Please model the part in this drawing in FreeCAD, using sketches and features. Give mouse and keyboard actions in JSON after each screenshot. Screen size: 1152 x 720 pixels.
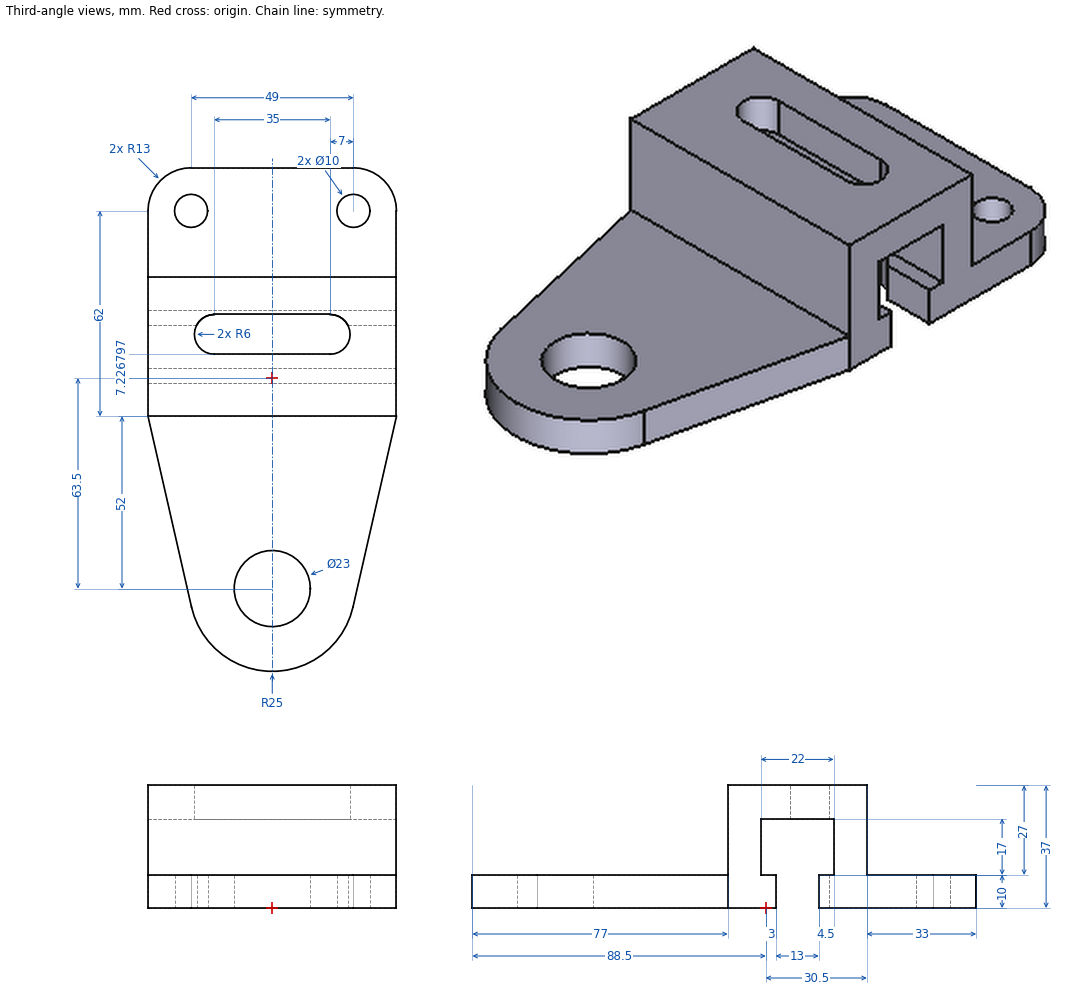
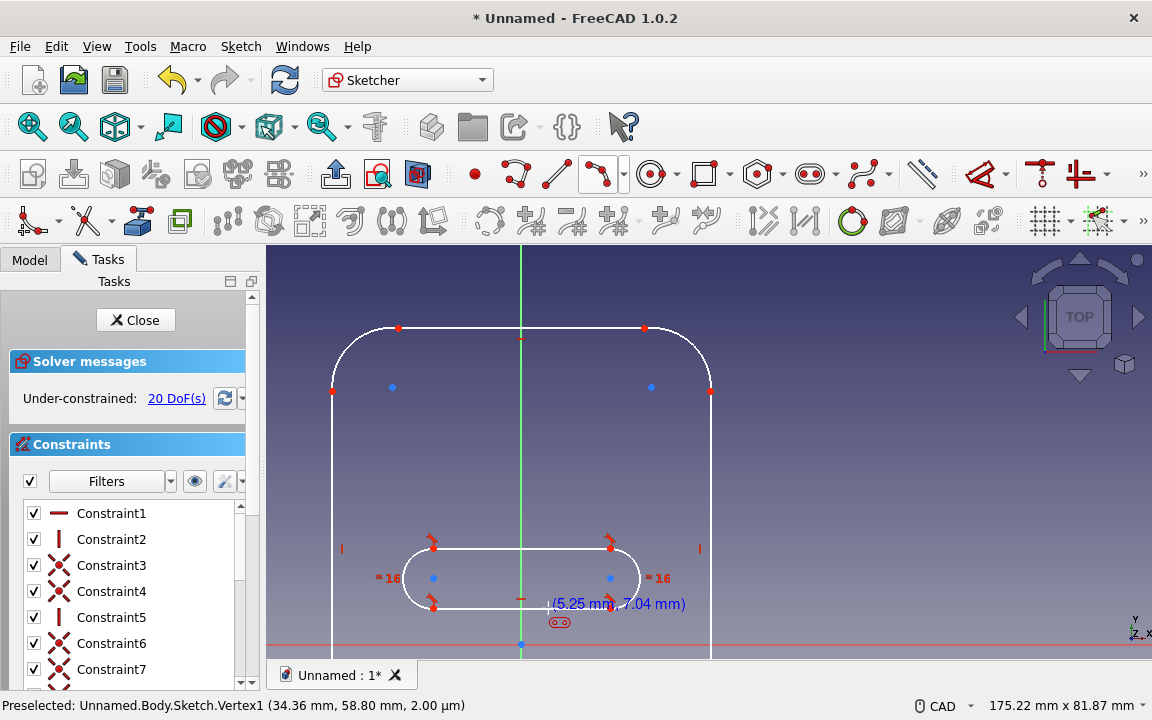
{"action": "left_click", "coordinate": [650, 174]}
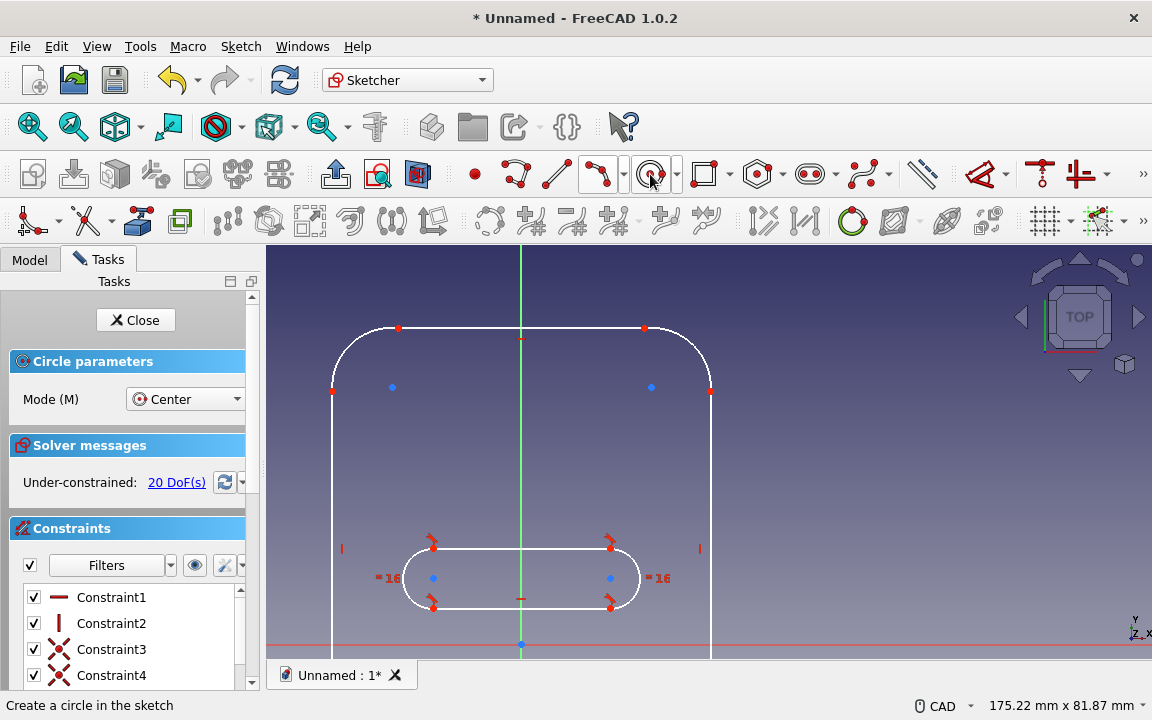
{"action": "scroll", "coordinate": [692, 342], "scroll_direction": "down", "scroll_amount": 6}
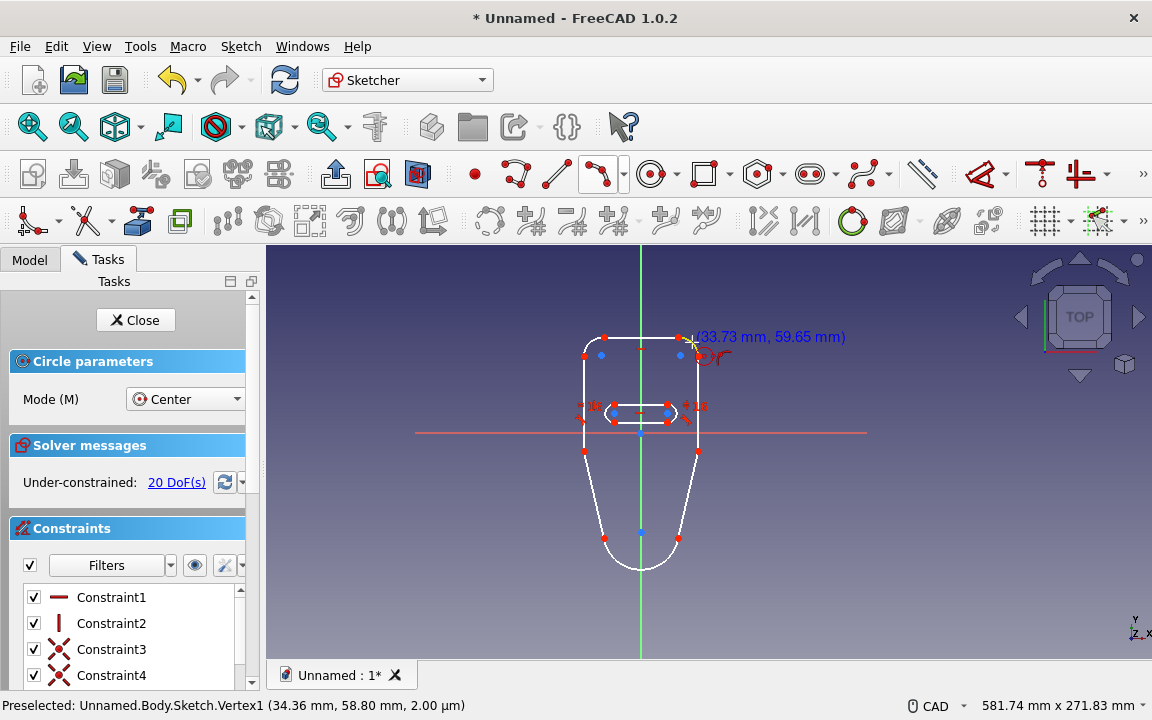
{"action": "scroll", "coordinate": [641, 530], "scroll_direction": "up", "scroll_amount": 2}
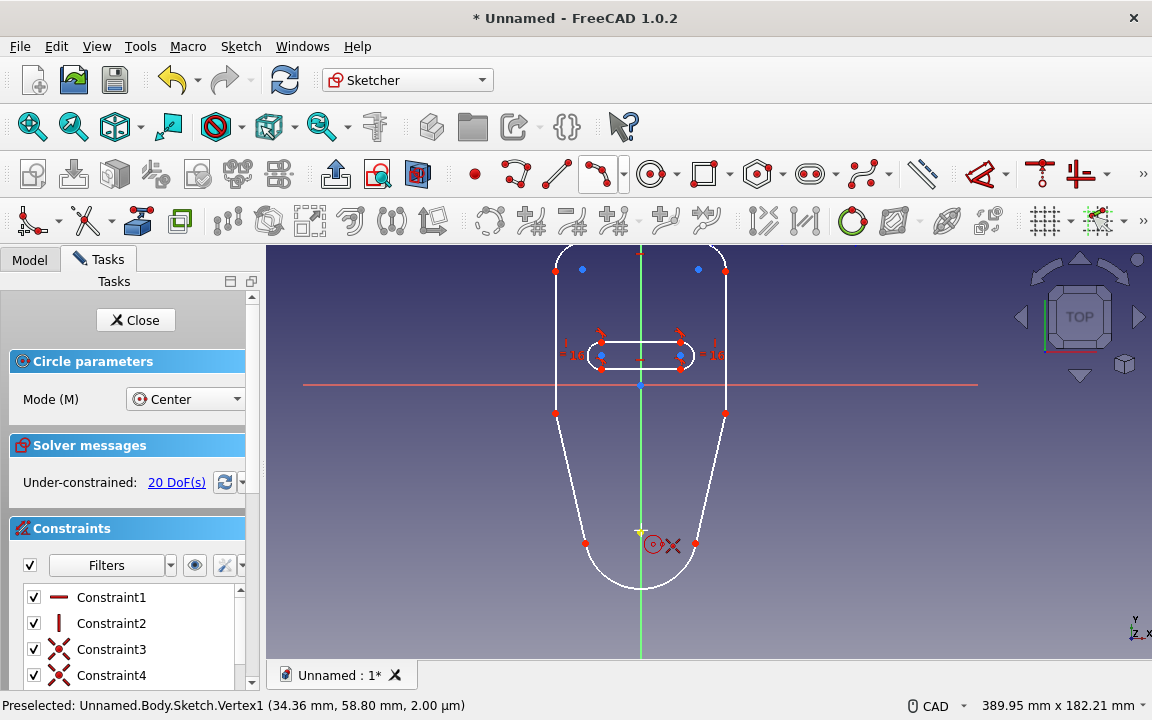
{"action": "left_click", "coordinate": [641, 530]}
{"action": "mouse_move", "coordinate": [659, 511]}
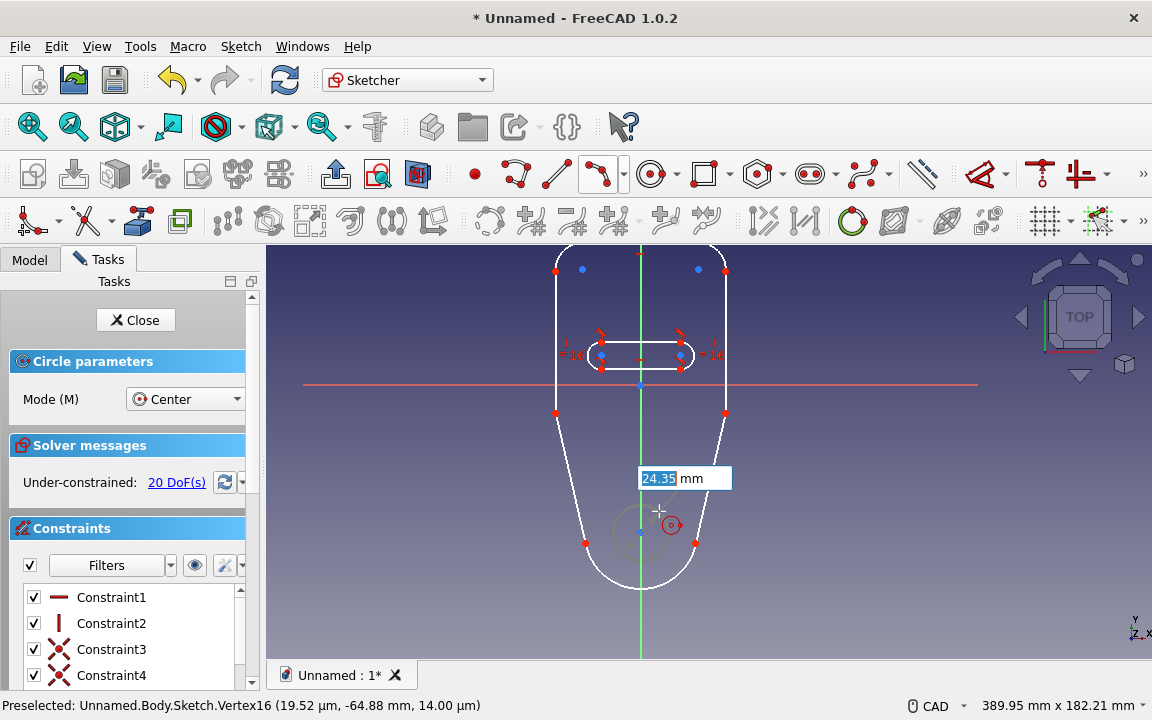
{"action": "type", "text": "23"}
{"action": "key", "text": "Return"}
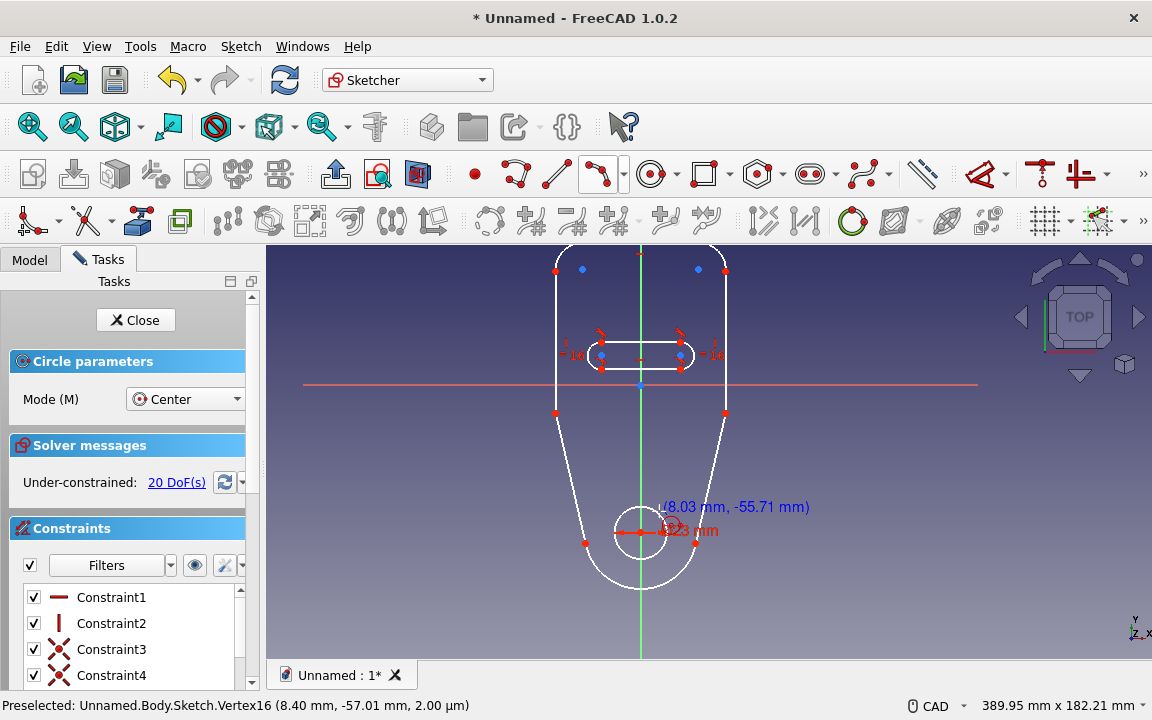
{"action": "scroll", "coordinate": [640, 530], "scroll_direction": "down", "scroll_amount": 2}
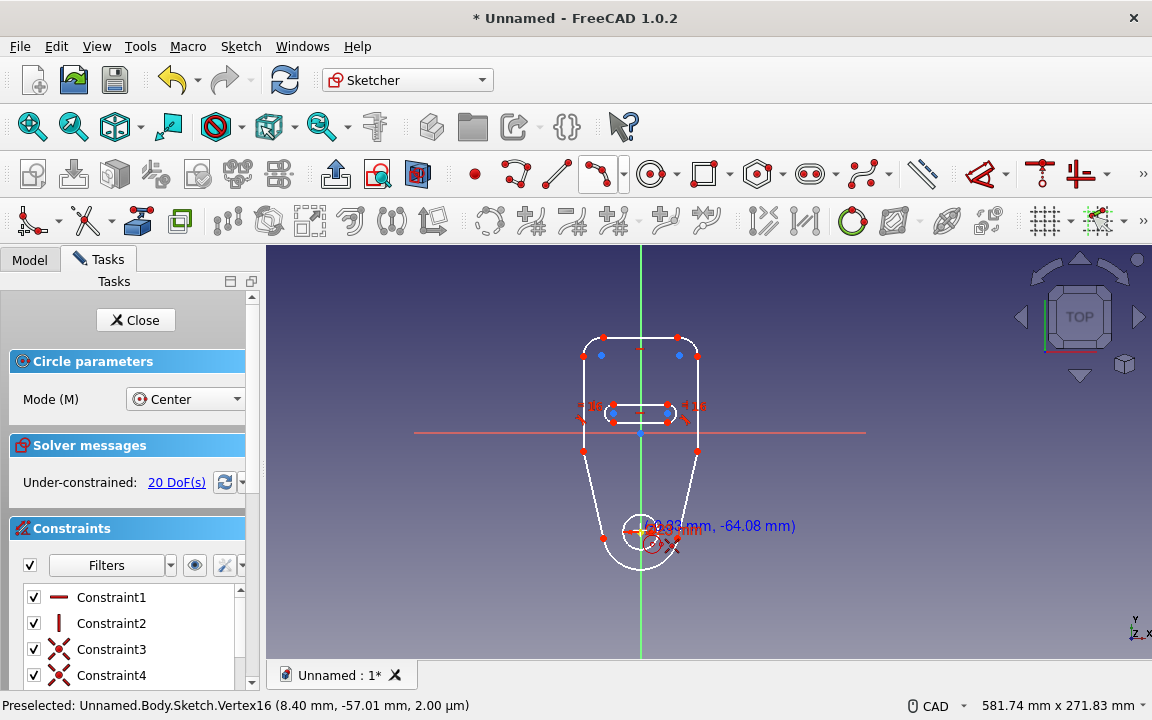
{"action": "scroll", "coordinate": [678, 356], "scroll_direction": "up", "scroll_amount": 6}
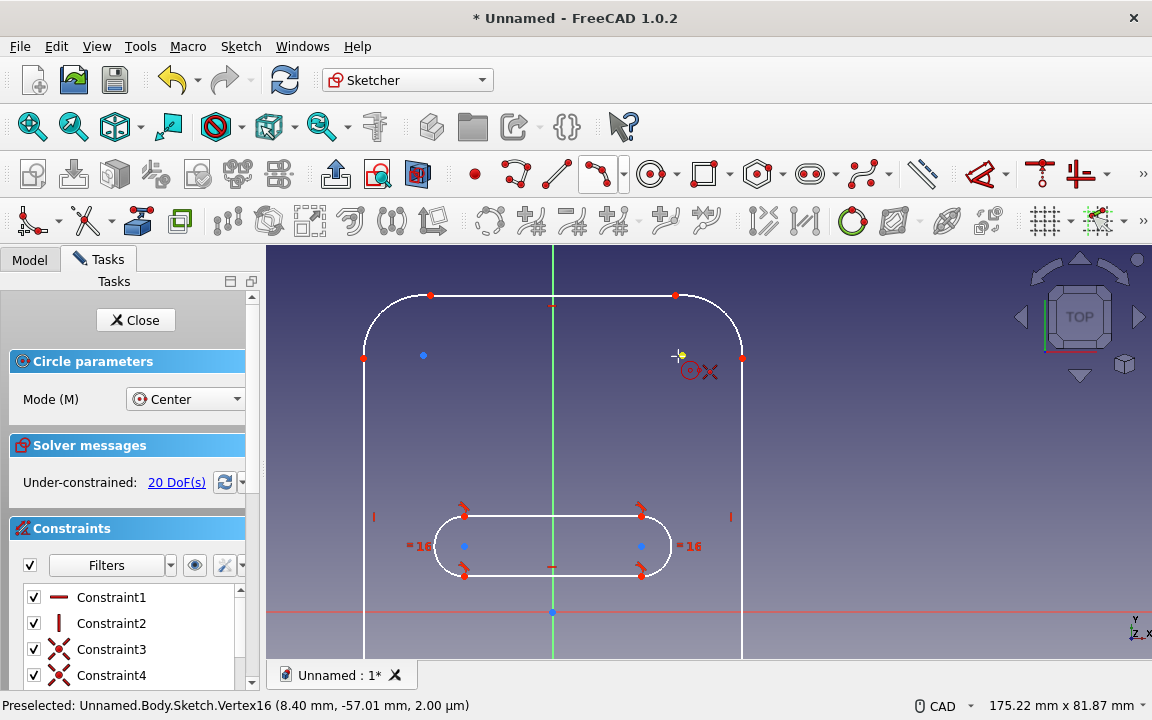
{"action": "left_click", "coordinate": [677, 357]}
{"action": "mouse_move", "coordinate": [695, 339]}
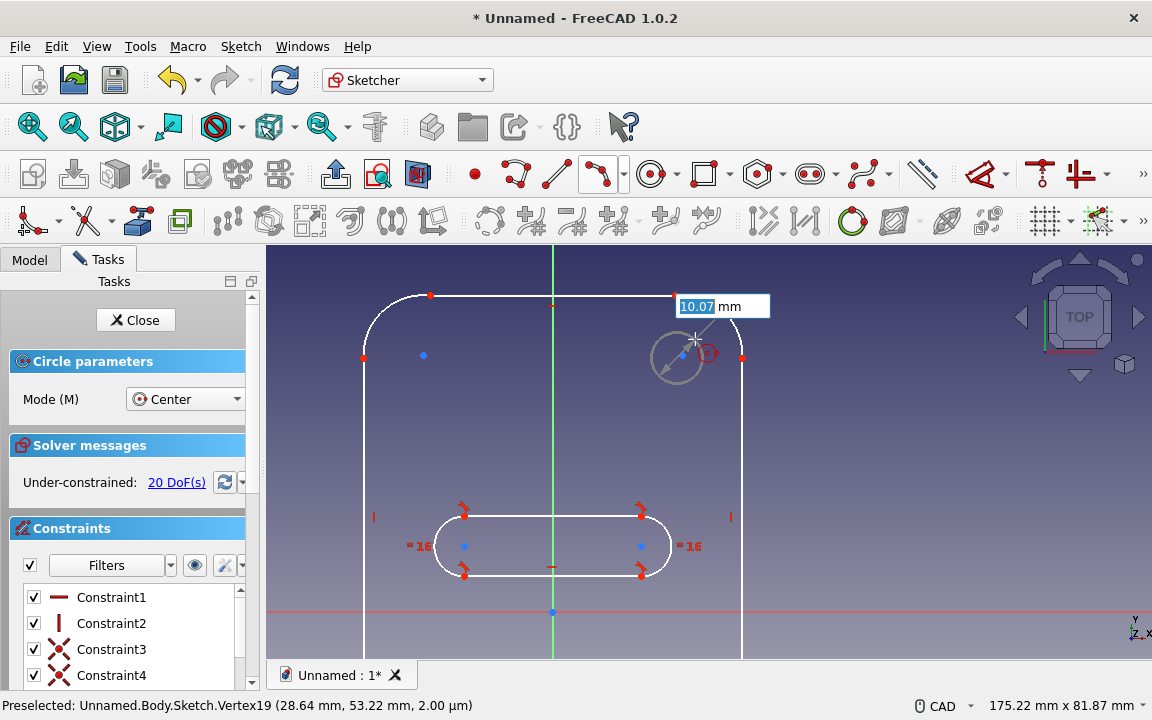
{"action": "type", "text": "10"}
{"action": "key", "text": "Return"}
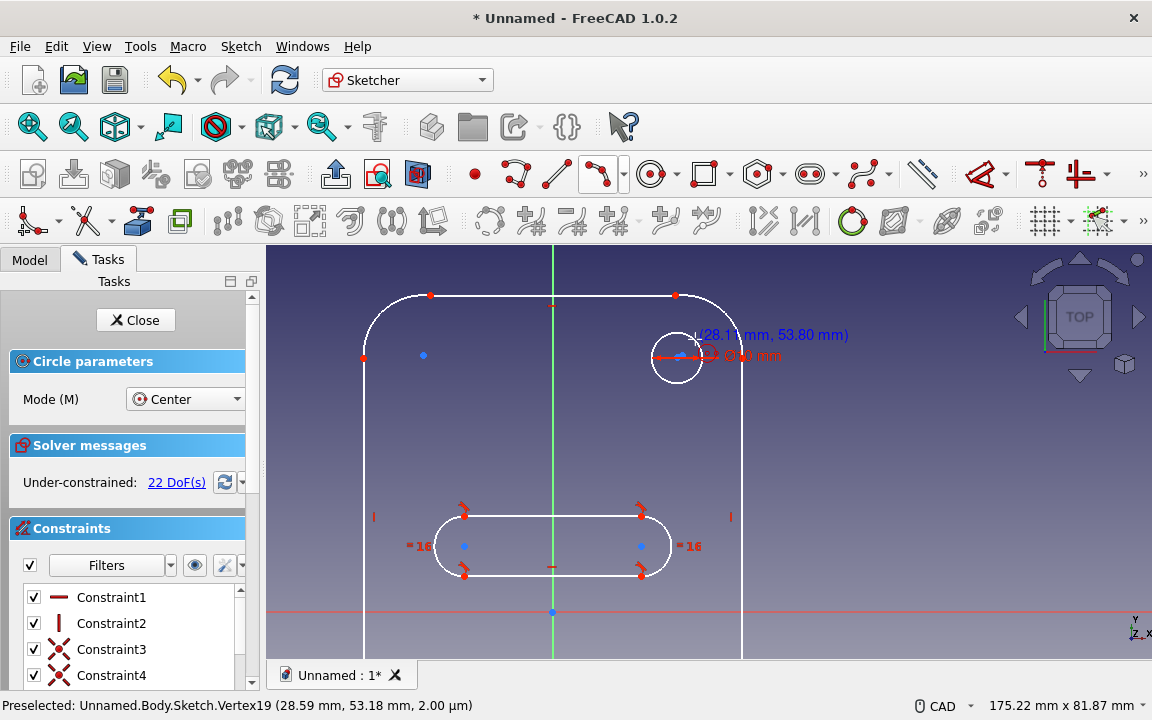
{"action": "left_click", "coordinate": [429, 357]}
{"action": "mouse_move", "coordinate": [447, 339]}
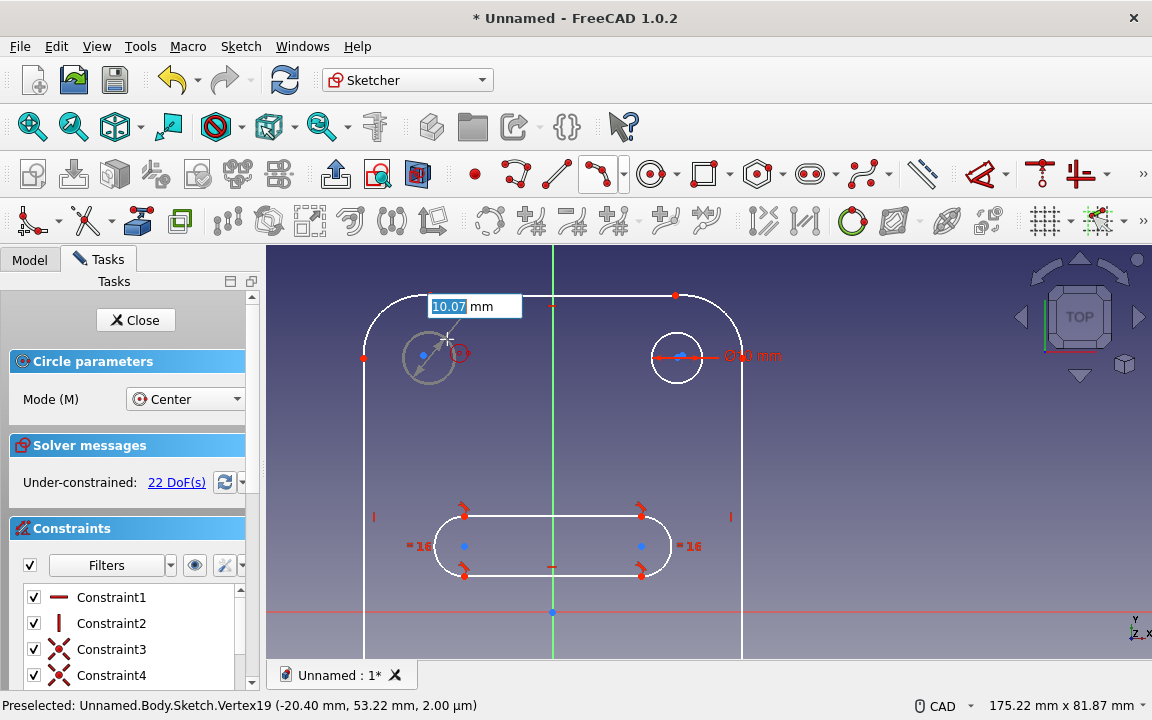
{"action": "type", "text": "10"}
{"action": "key", "text": "Return"}
{"action": "key", "text": "Escape"}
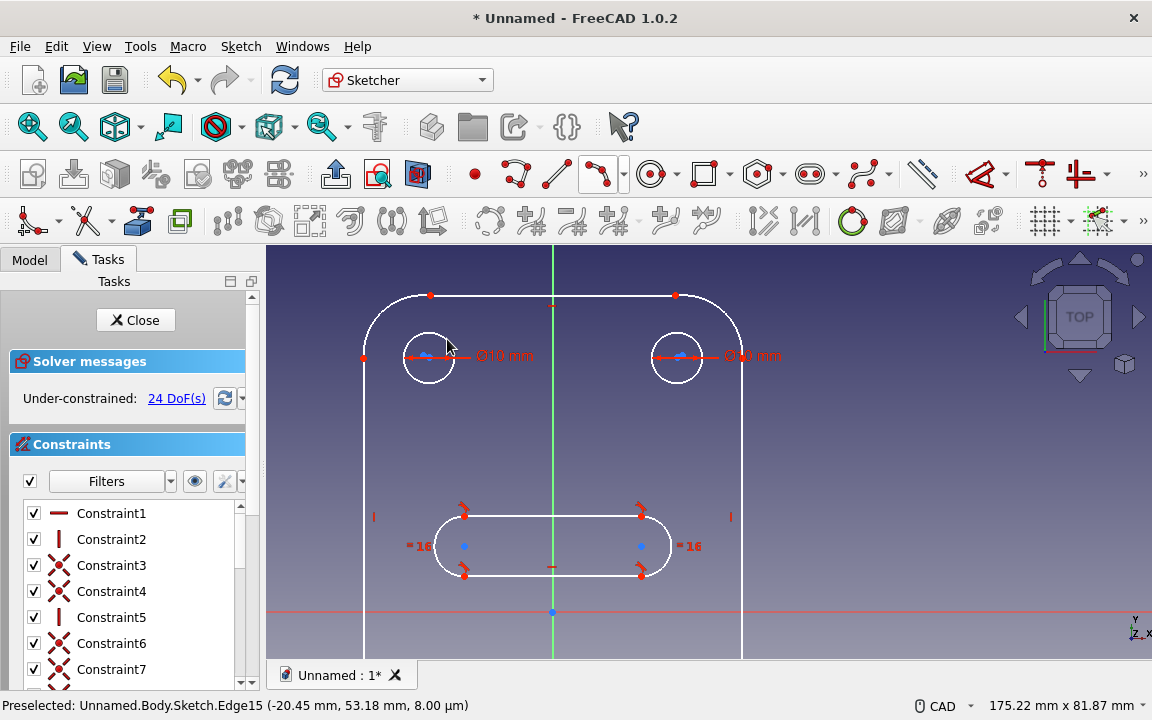
{"action": "left_click", "coordinate": [602, 296]}